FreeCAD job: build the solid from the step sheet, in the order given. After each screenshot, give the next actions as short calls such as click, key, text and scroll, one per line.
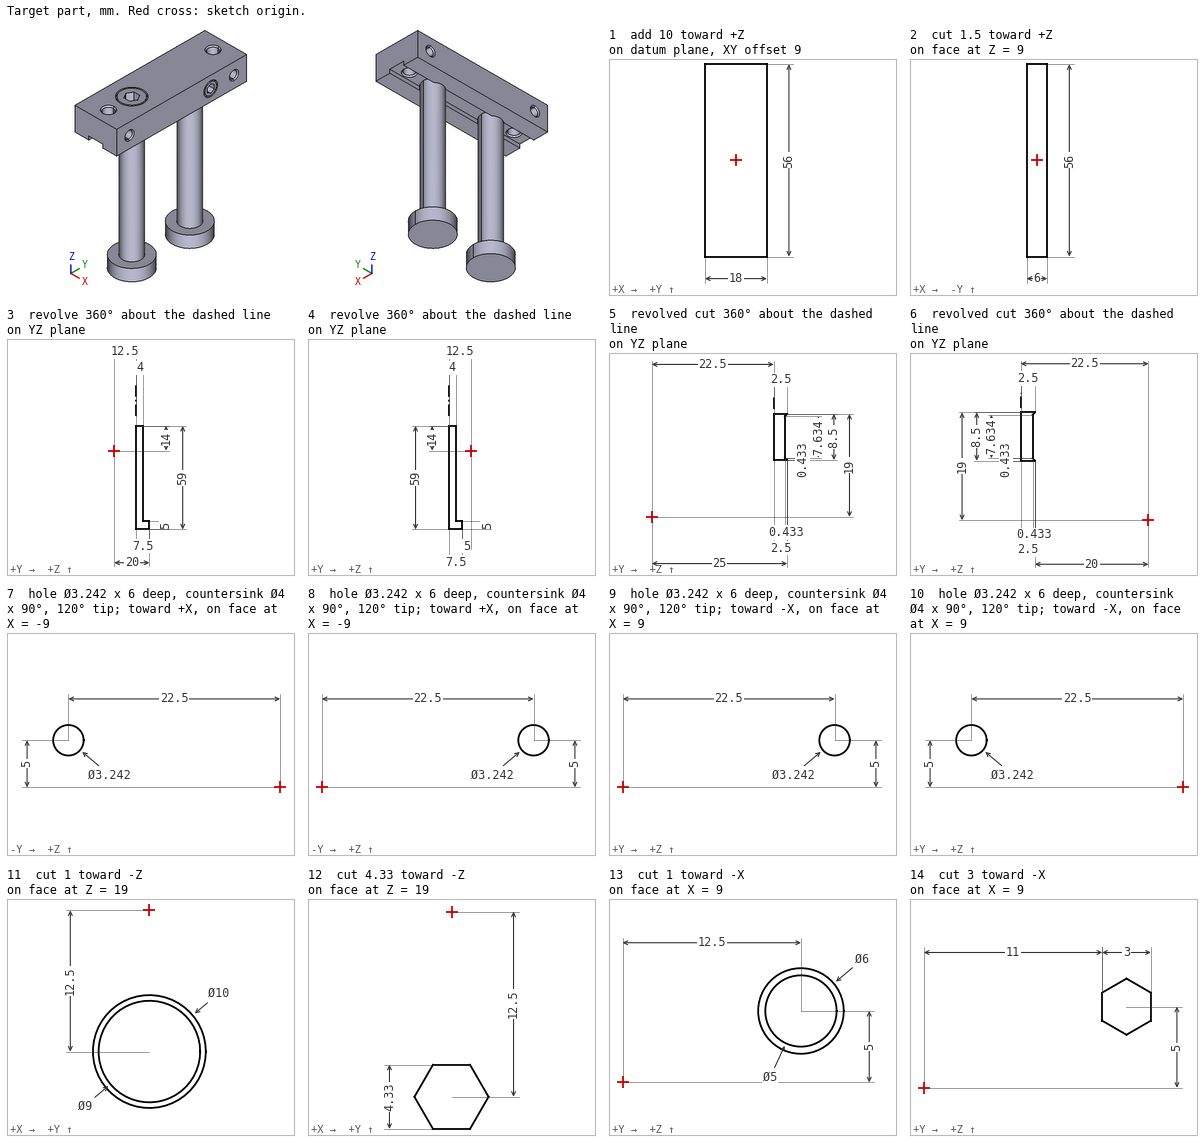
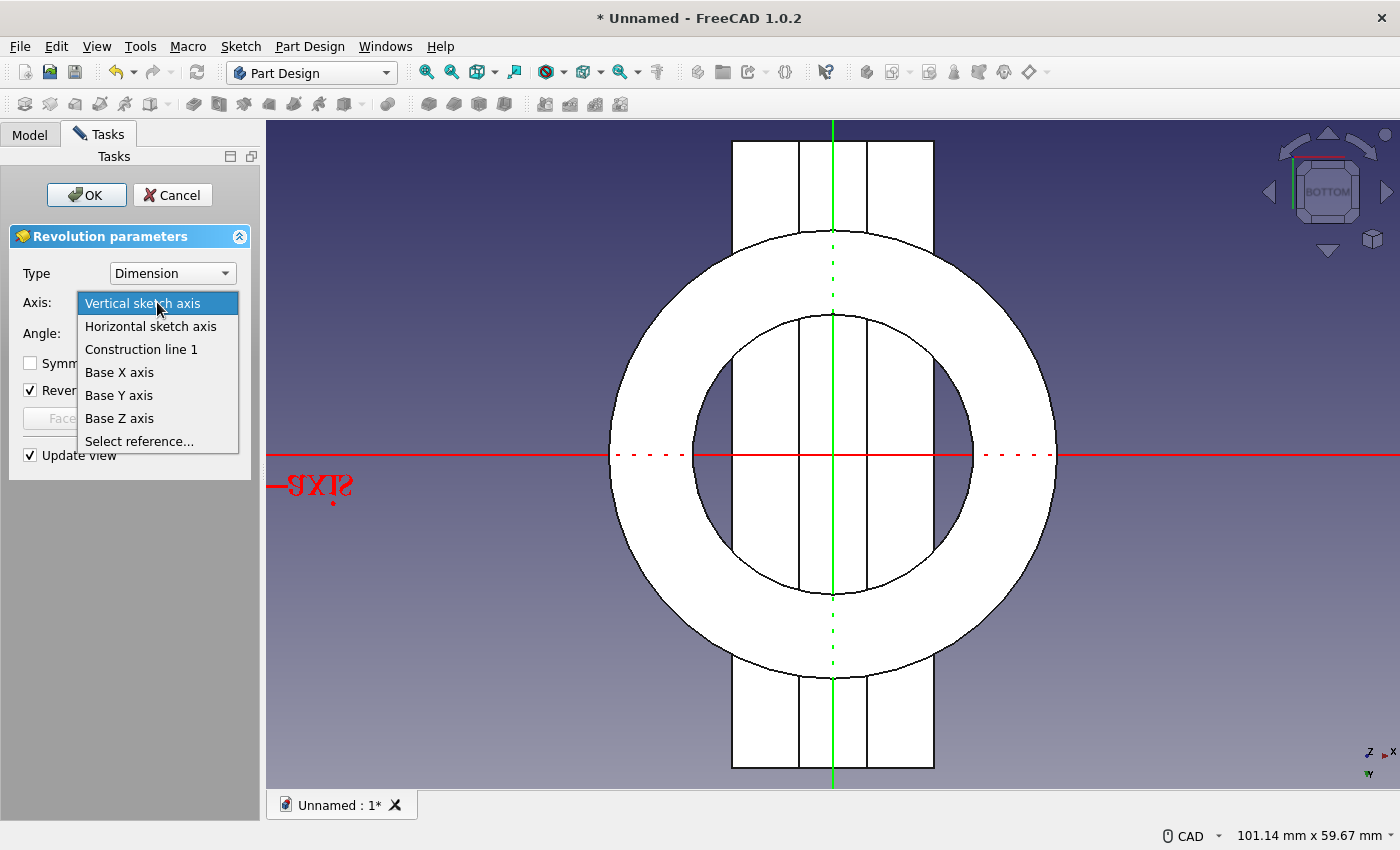
click(156, 350)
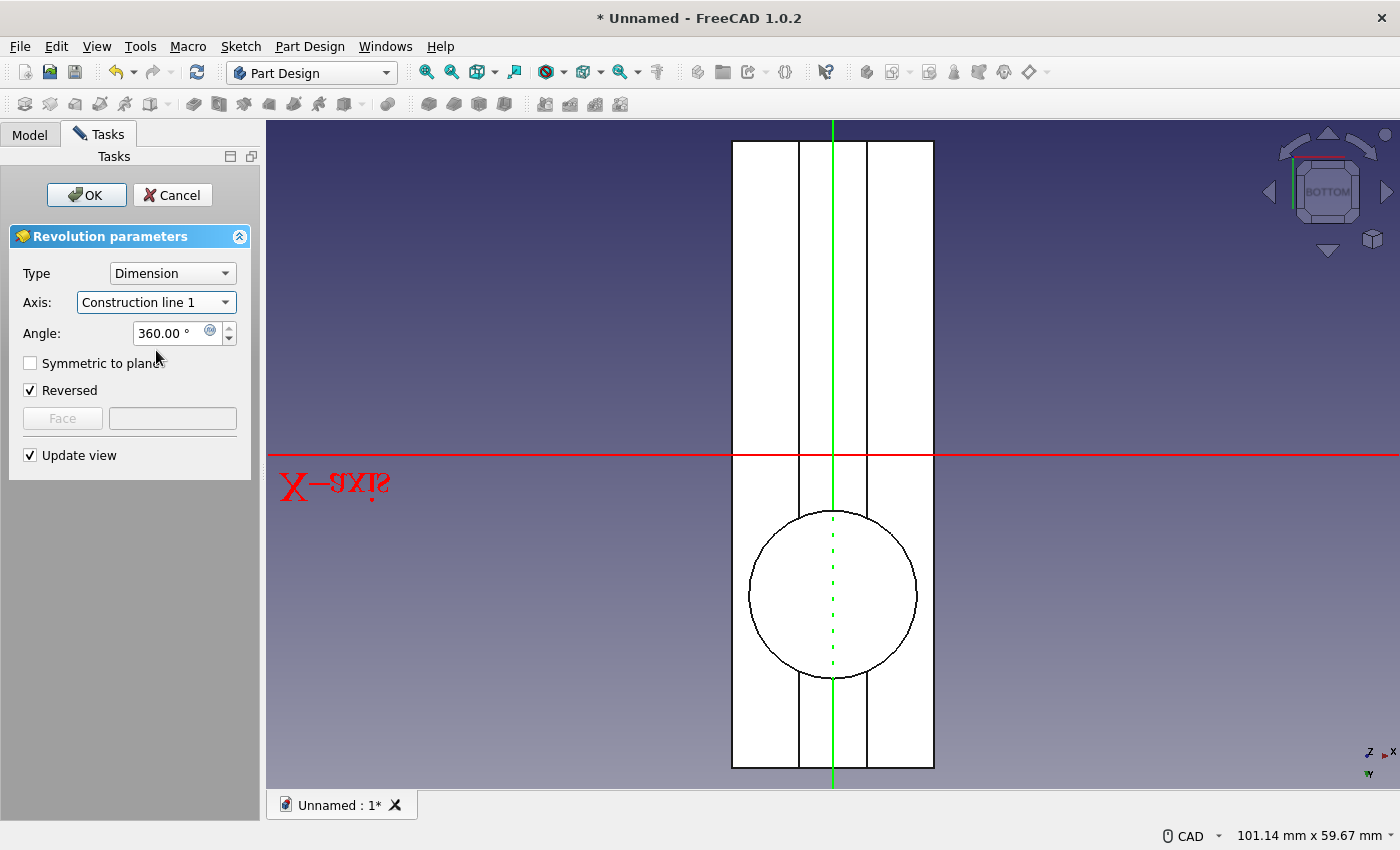
click(87, 195)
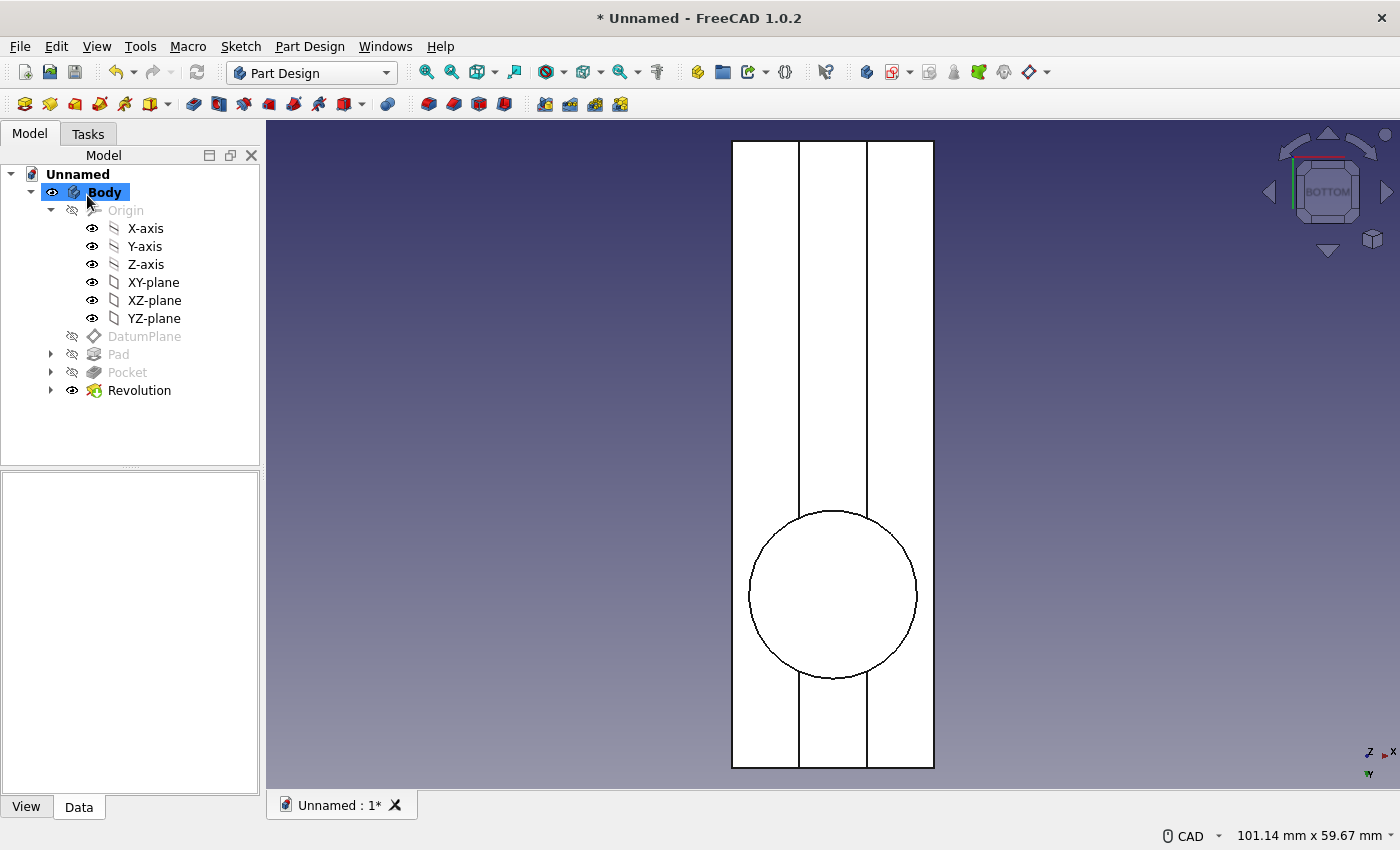
click(892, 72)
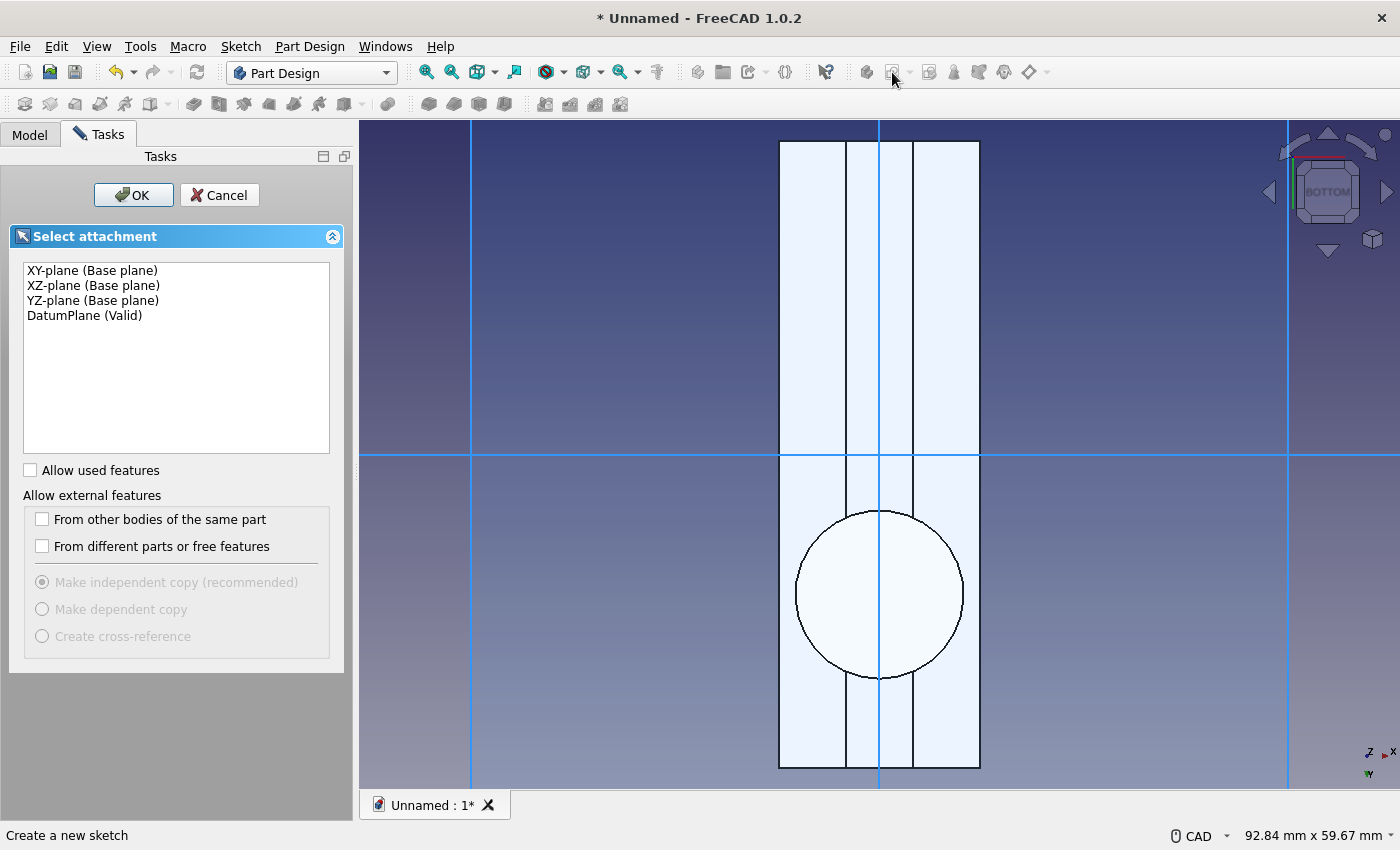
click(84, 300)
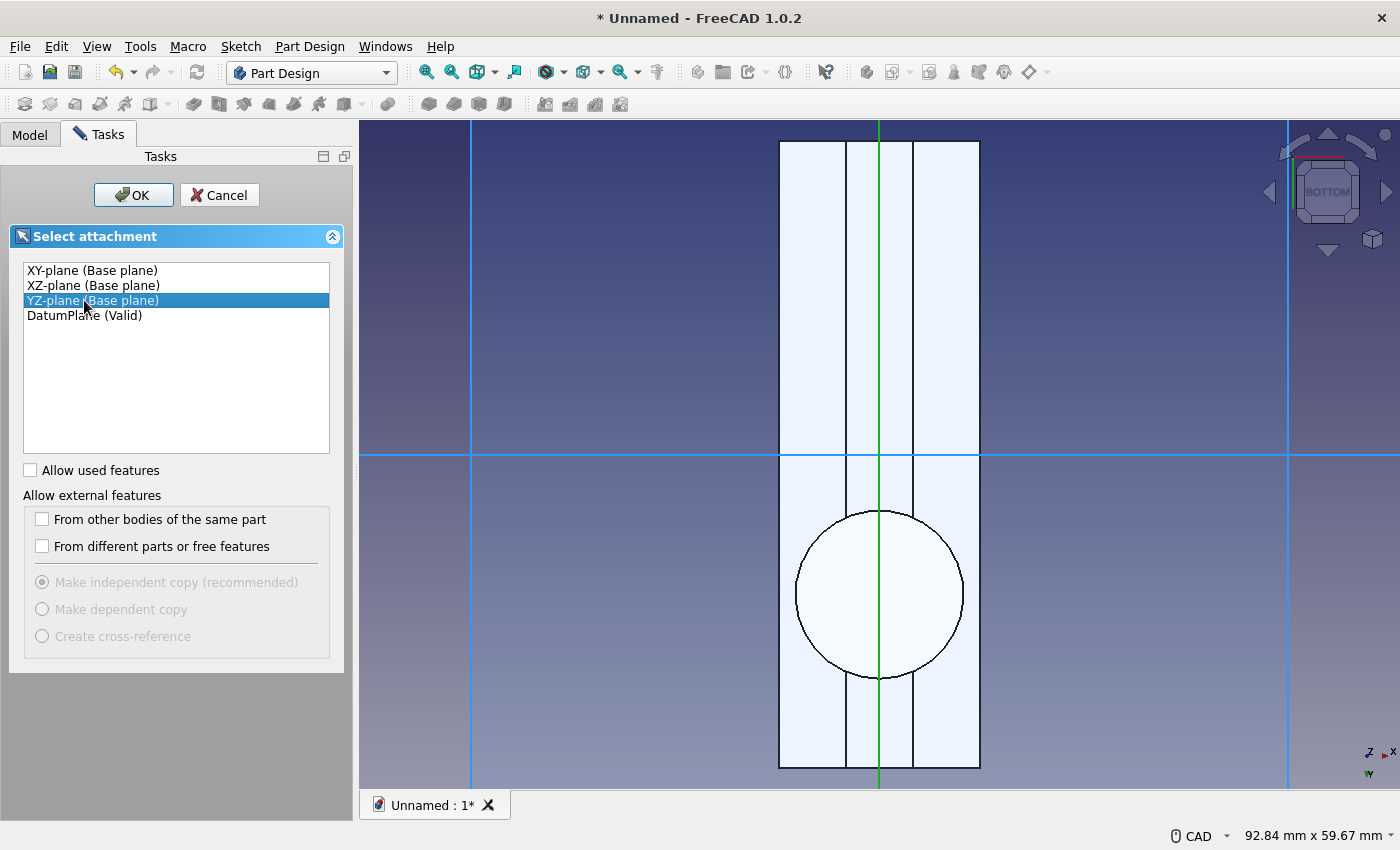
click(134, 195)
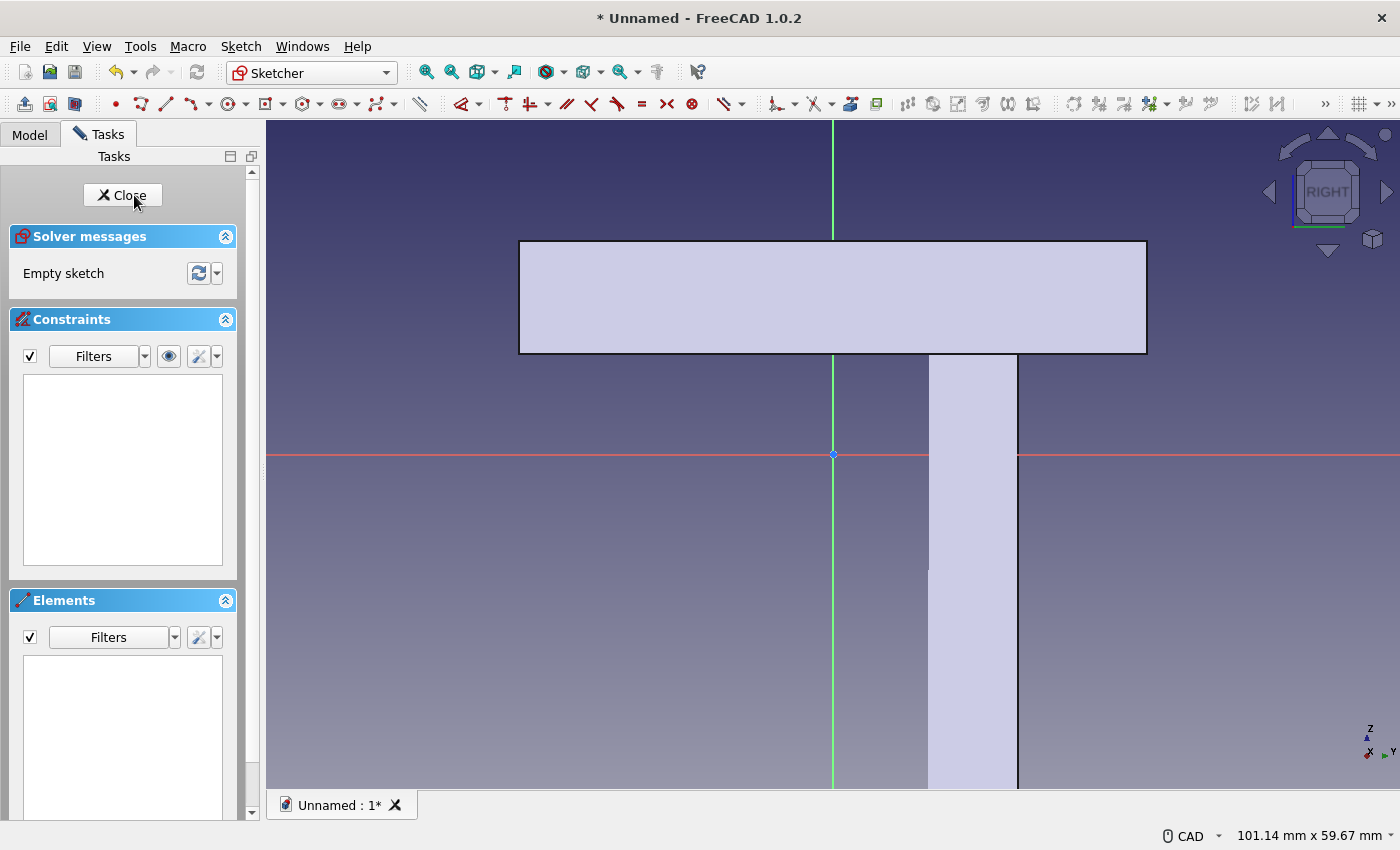
click(75, 104)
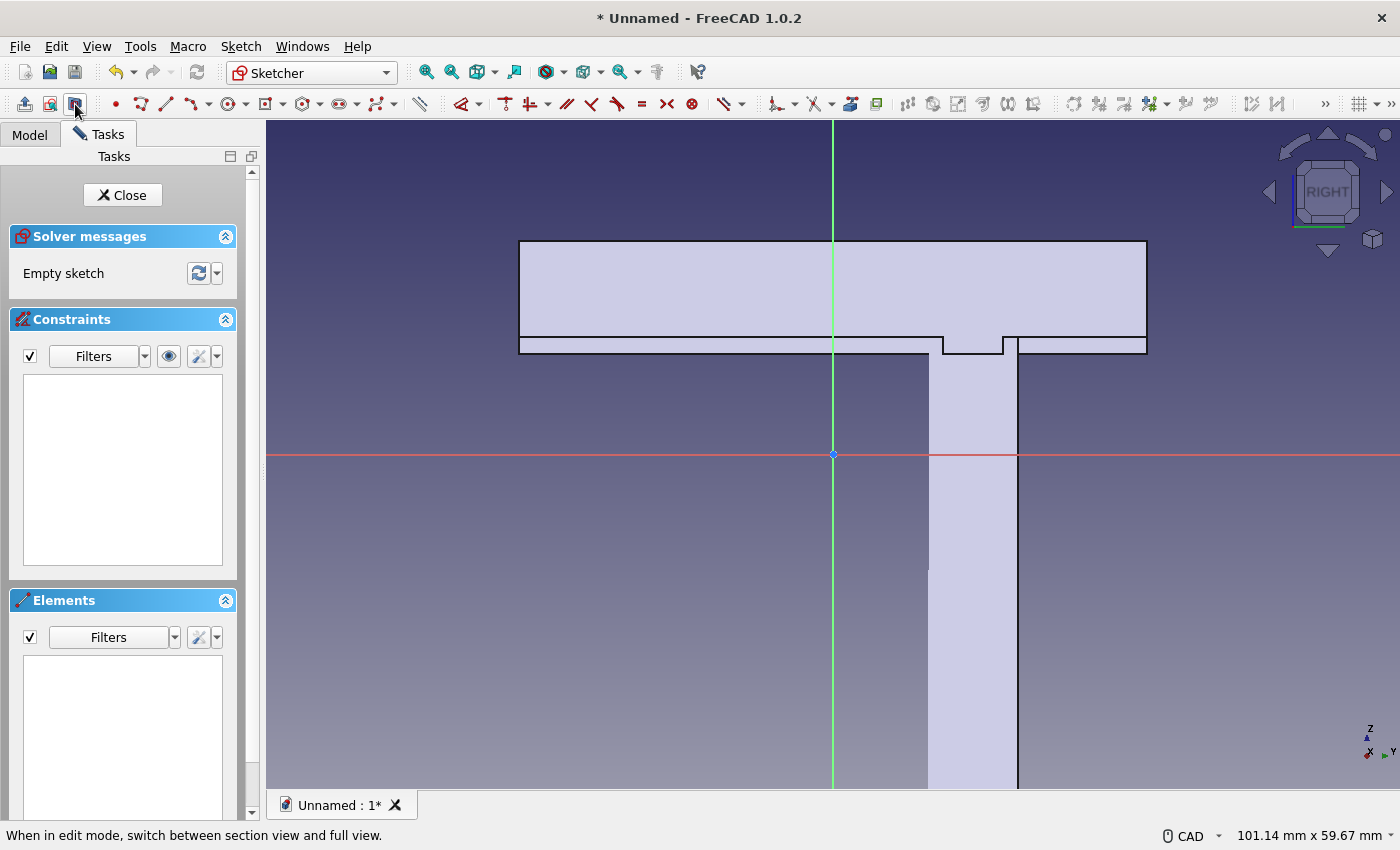
scroll(766, 421, down, 4)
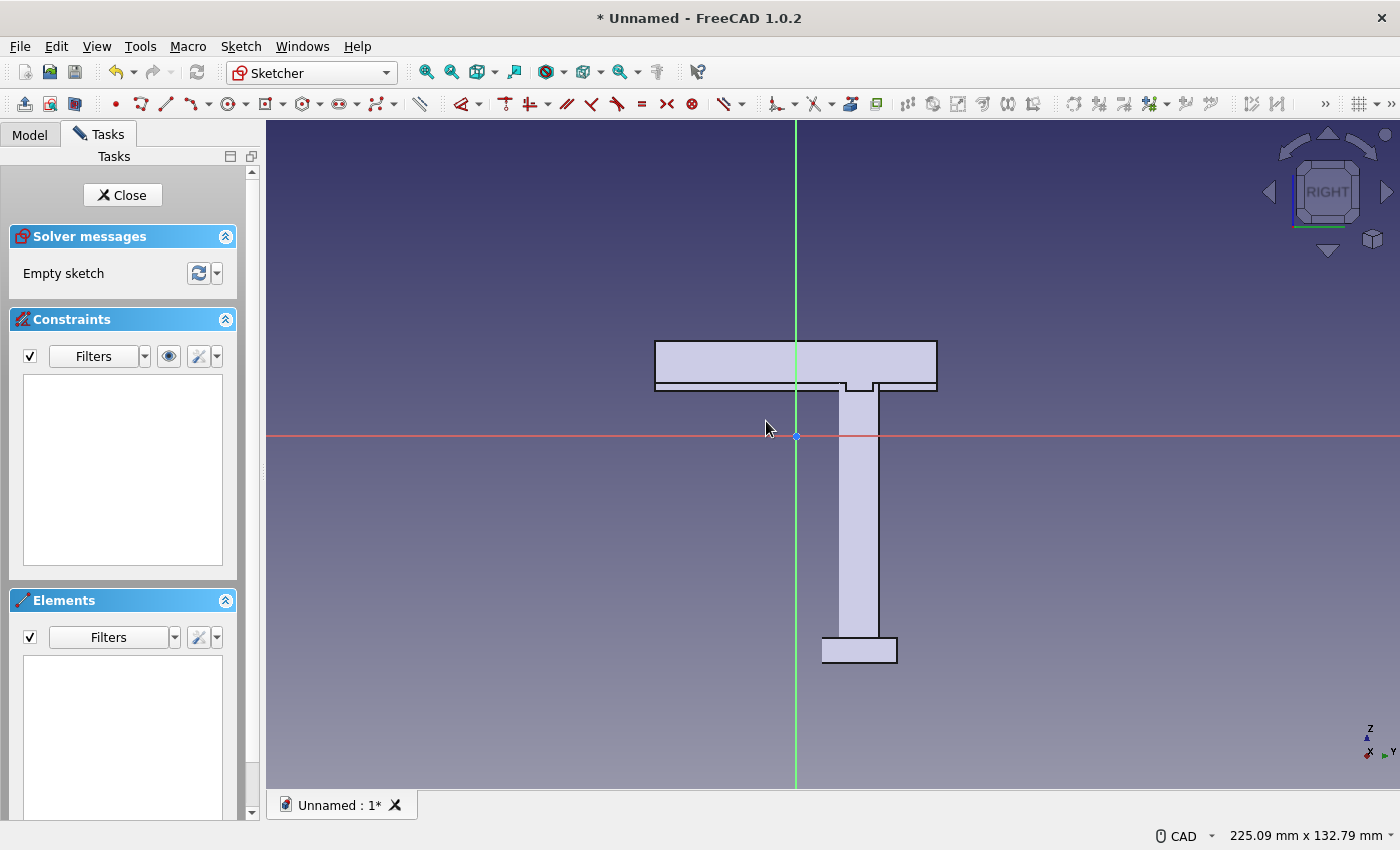
click(141, 104)